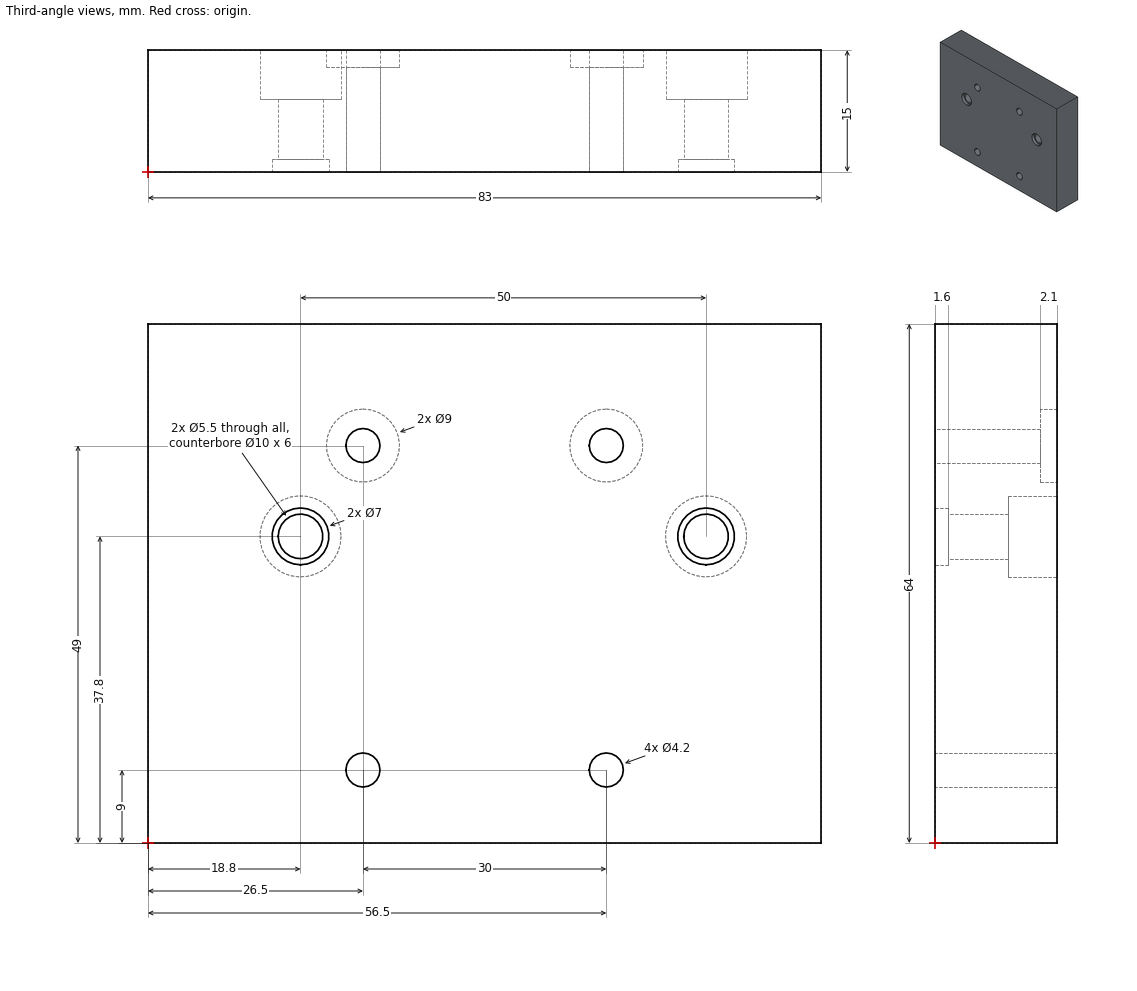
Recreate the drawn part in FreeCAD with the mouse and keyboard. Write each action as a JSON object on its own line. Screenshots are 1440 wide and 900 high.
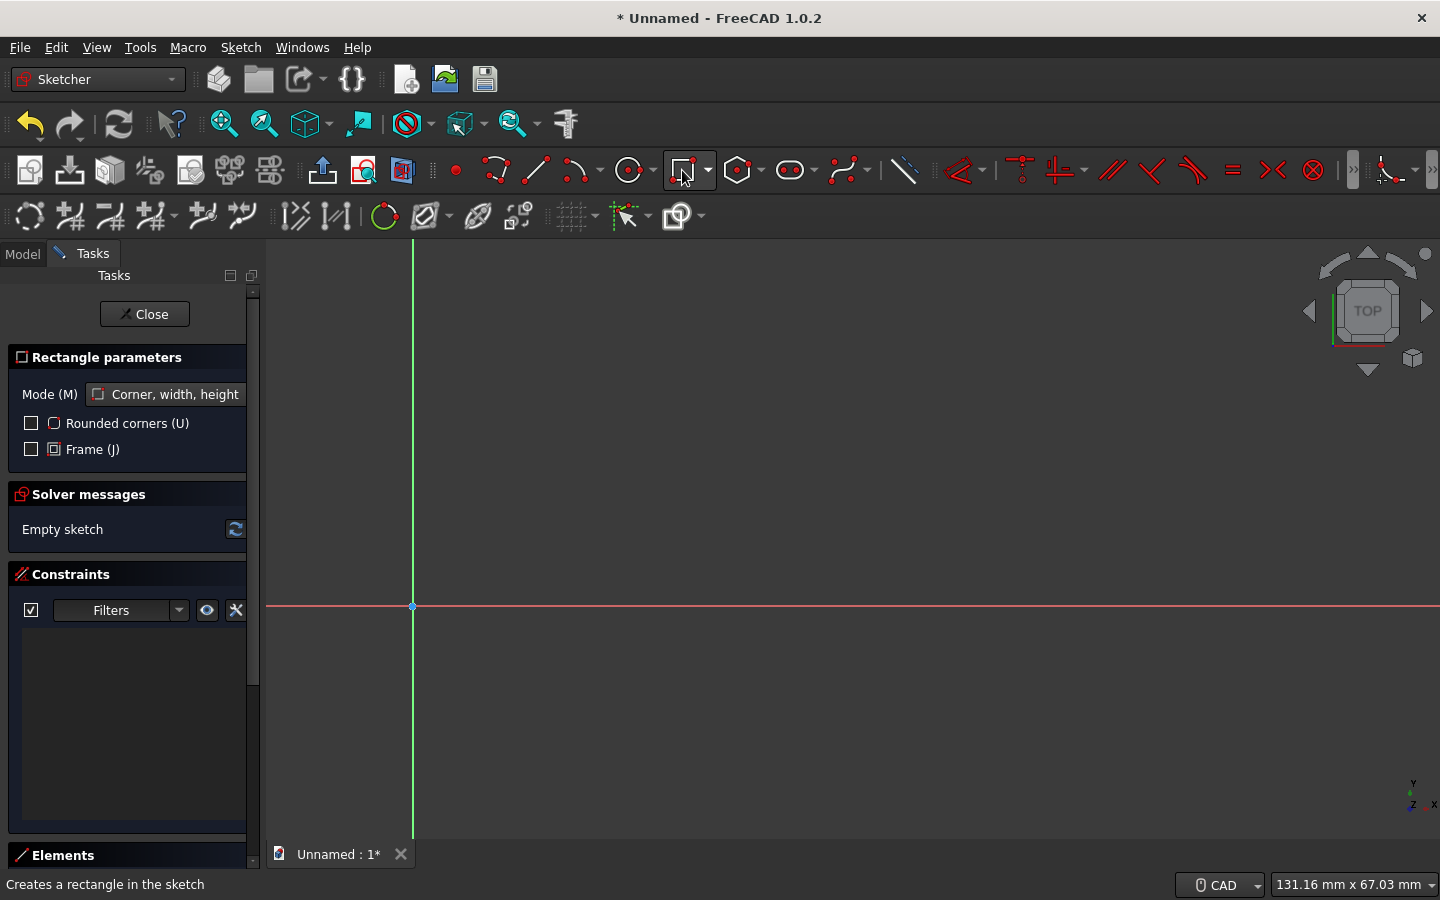
{"action": "left_click", "coordinate": [413, 606]}
{"action": "left_click", "coordinate": [1156, 472]}
{"action": "key", "text": "Escape"}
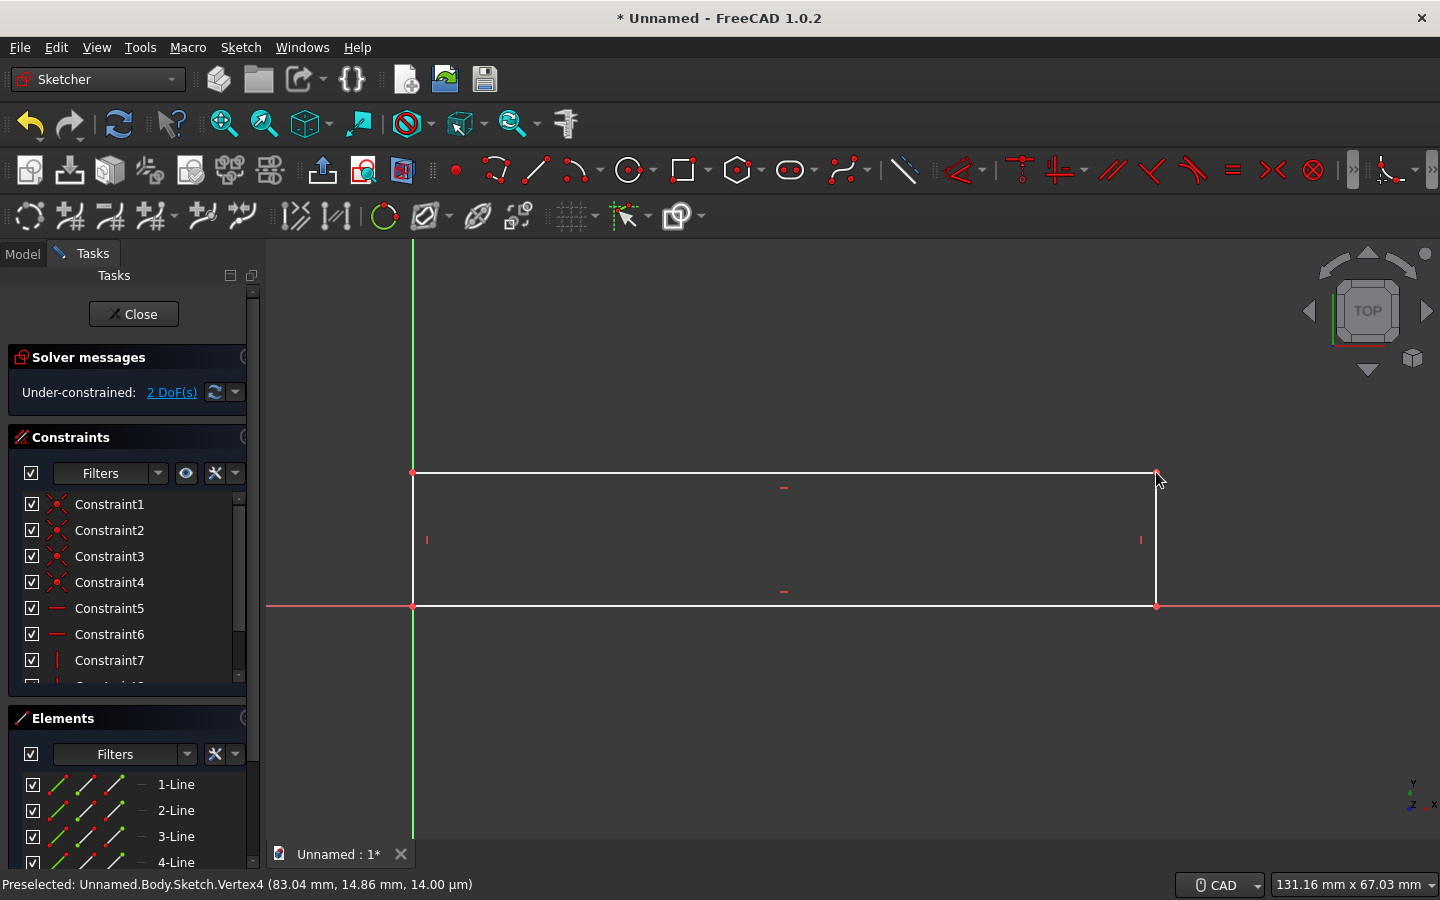
{"action": "left_click", "coordinate": [958, 170]}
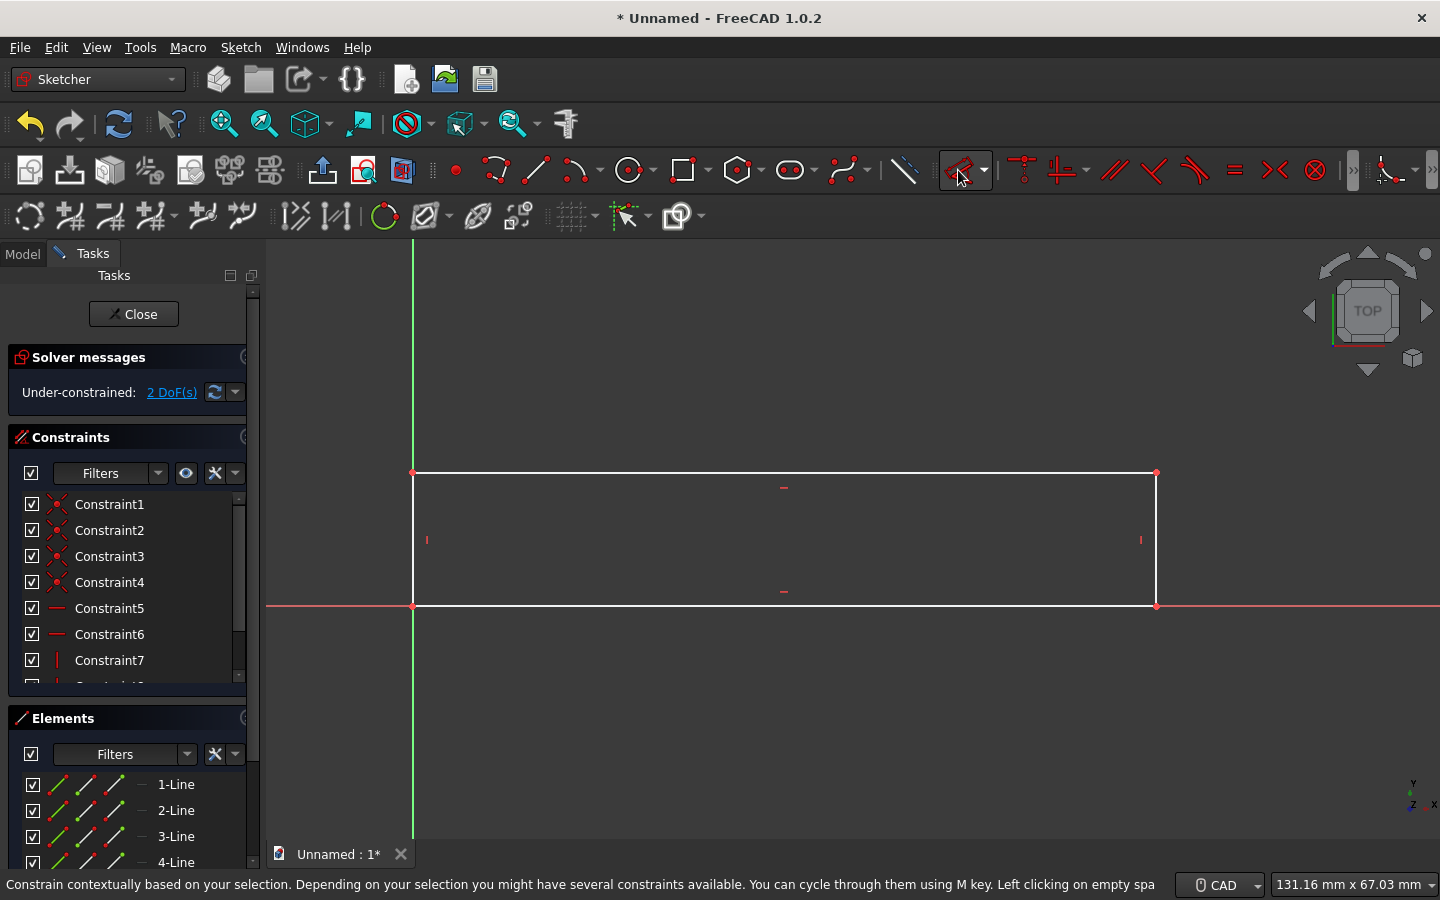
{"action": "left_click", "coordinate": [636, 606]}
{"action": "left_click", "coordinate": [784, 640]}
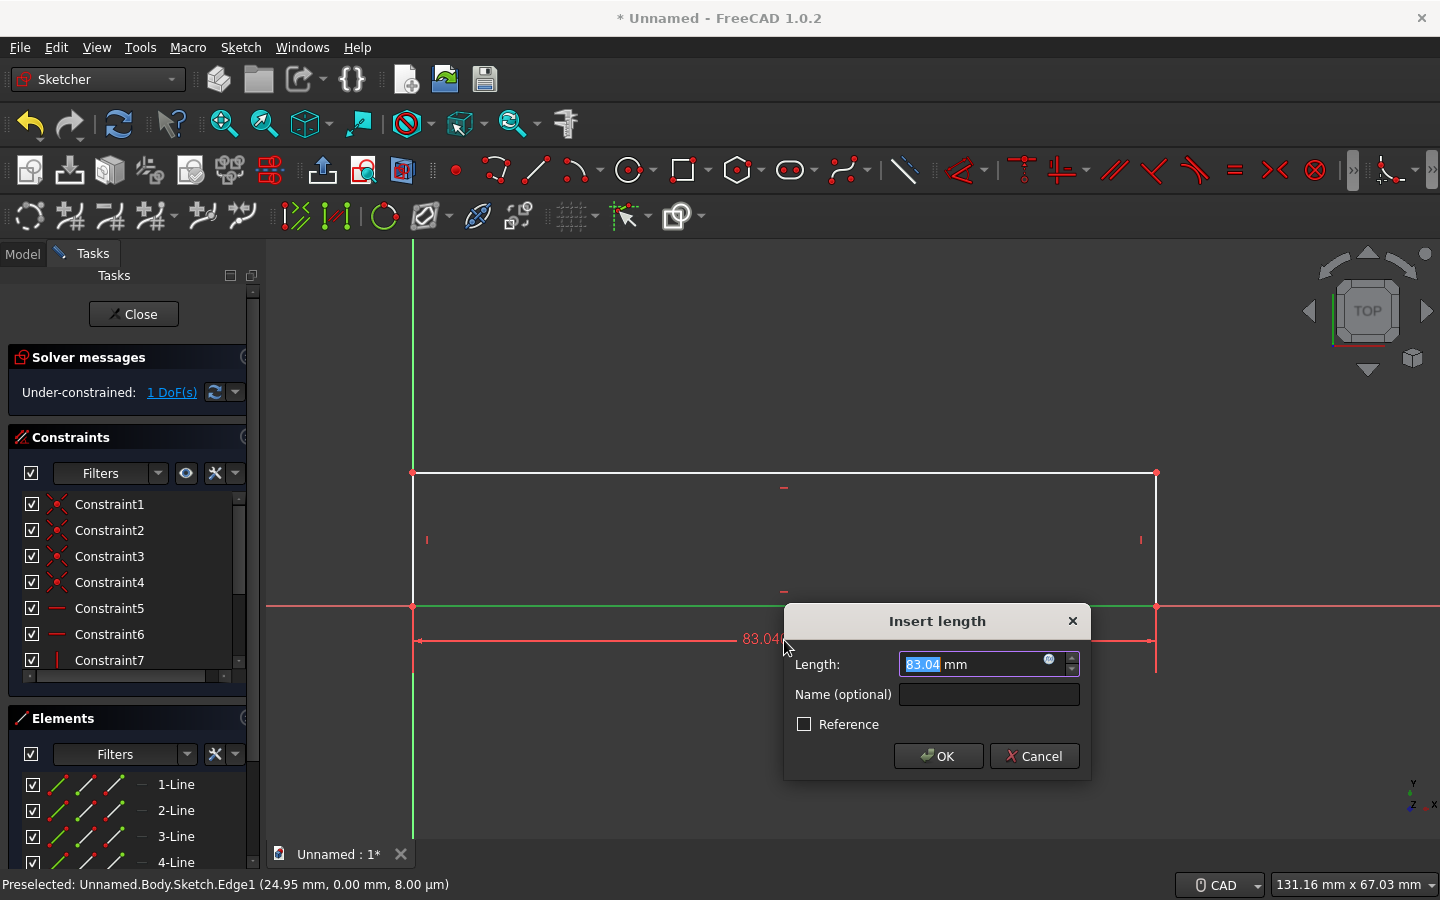
{"action": "type", "text": "83"}
{"action": "key", "text": "Return"}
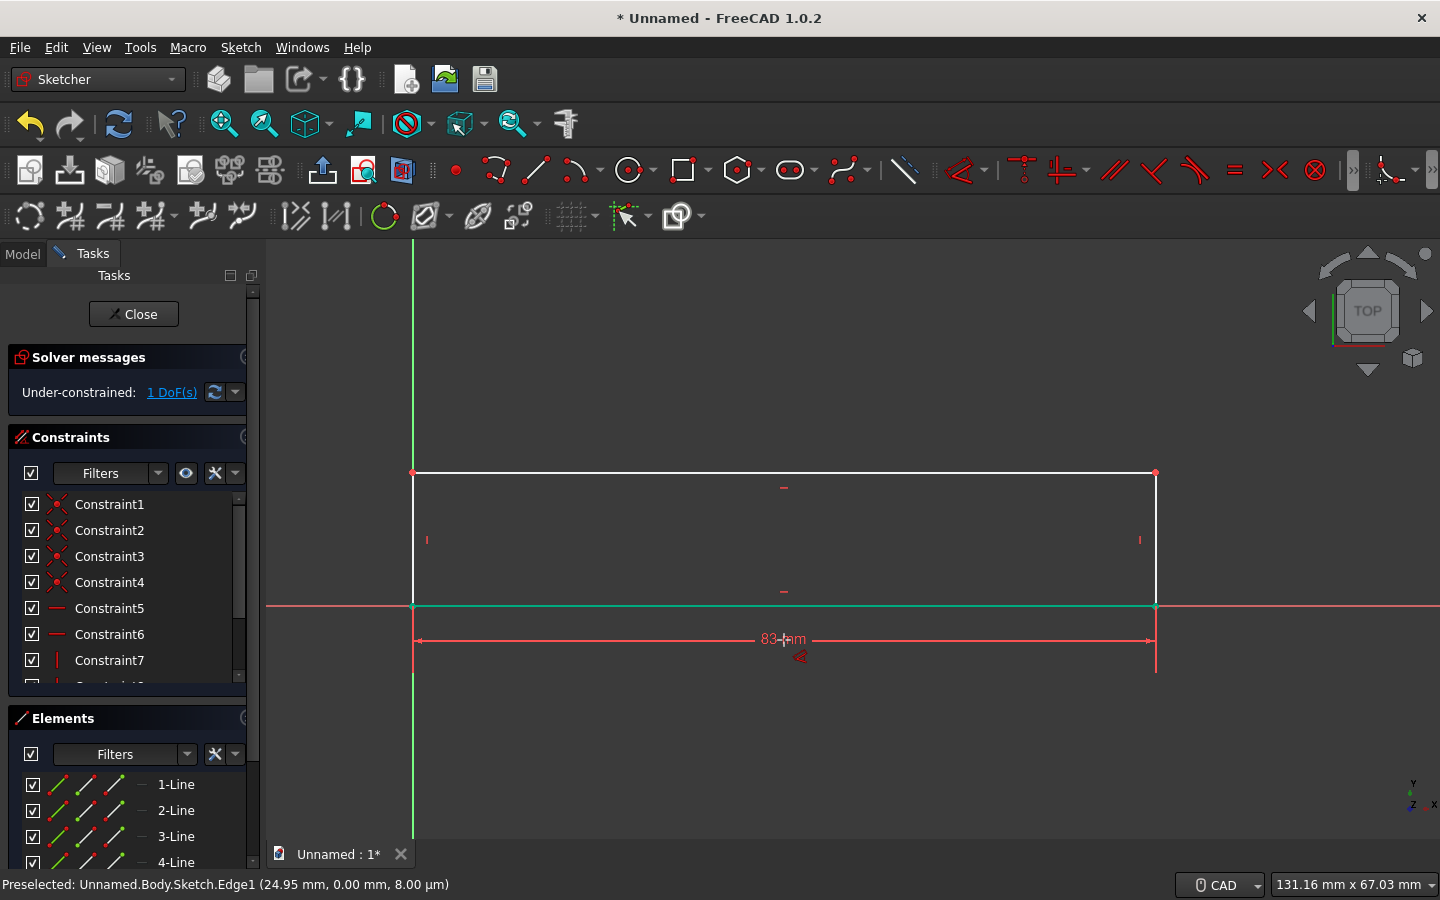
{"action": "left_click", "coordinate": [1156, 566]}
{"action": "left_click", "coordinate": [1190, 540]}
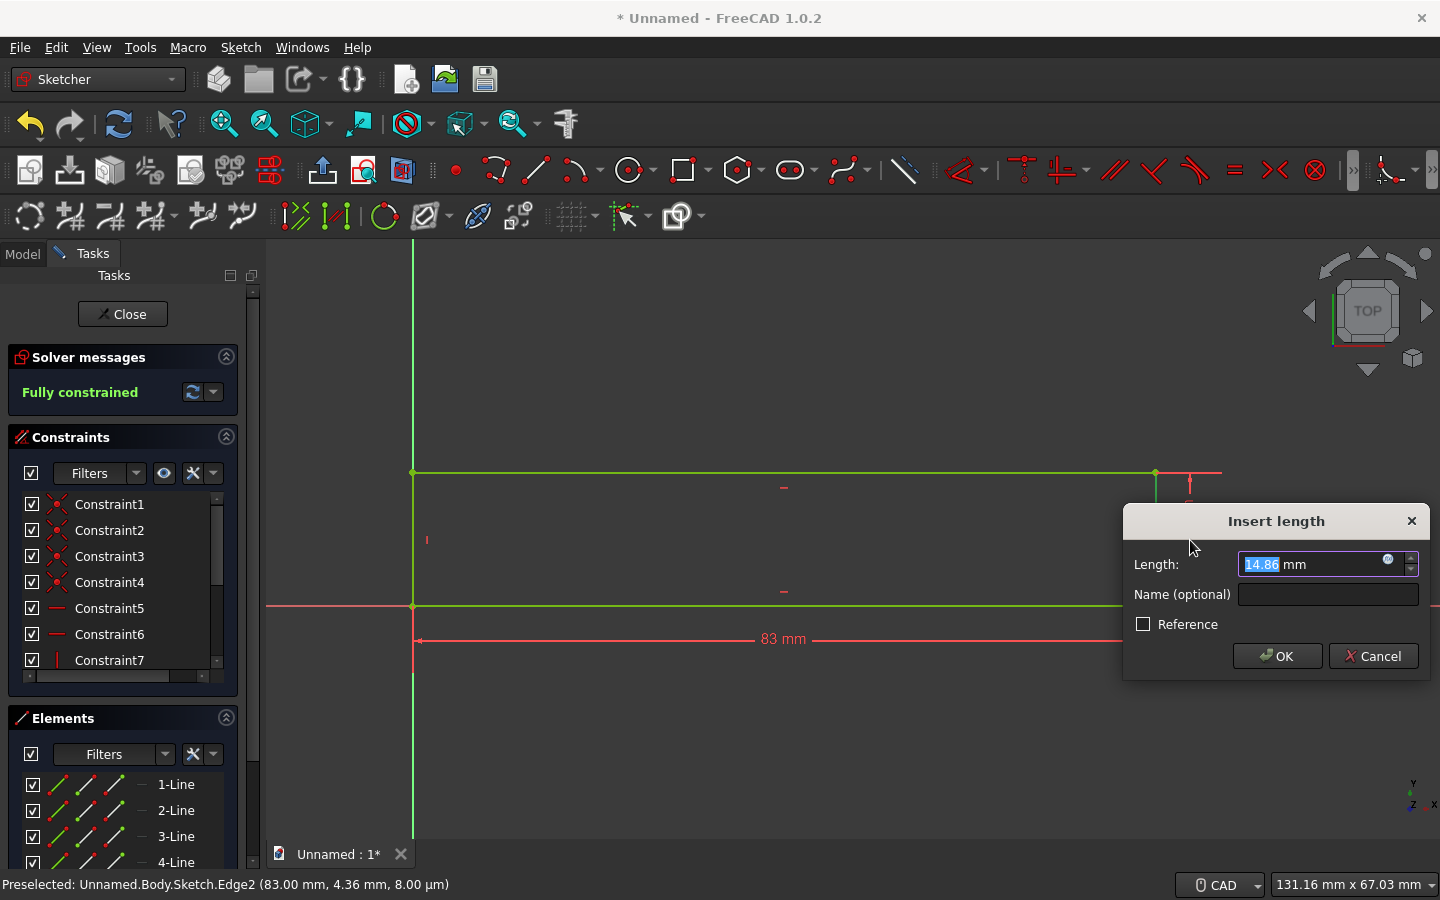
{"action": "type", "text": "15"}
{"action": "key", "text": "Return"}
{"action": "key", "text": "Escape"}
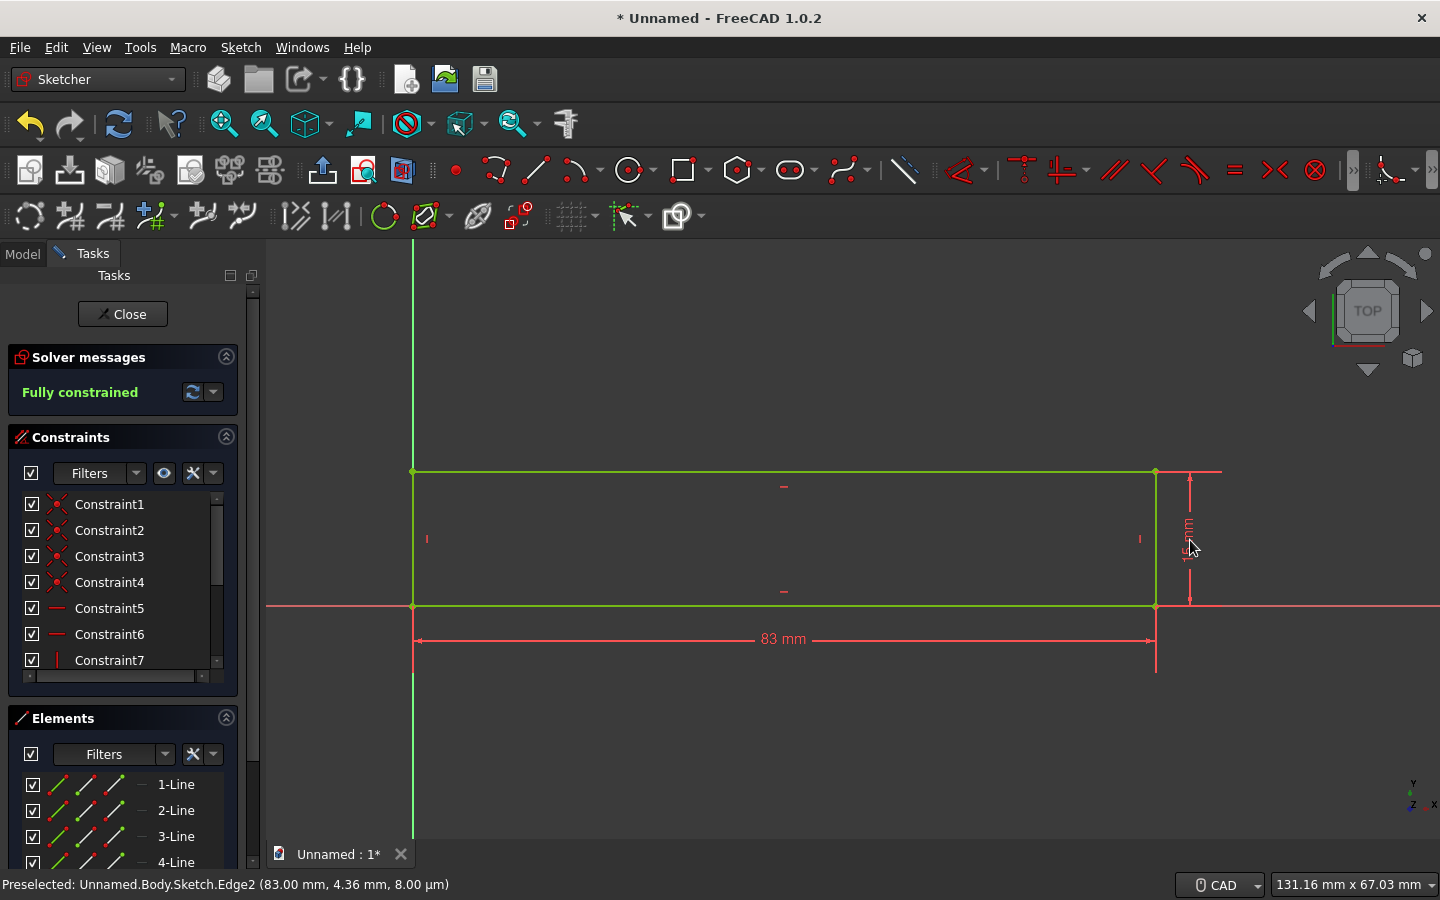
{"action": "left_click", "coordinate": [123, 314]}